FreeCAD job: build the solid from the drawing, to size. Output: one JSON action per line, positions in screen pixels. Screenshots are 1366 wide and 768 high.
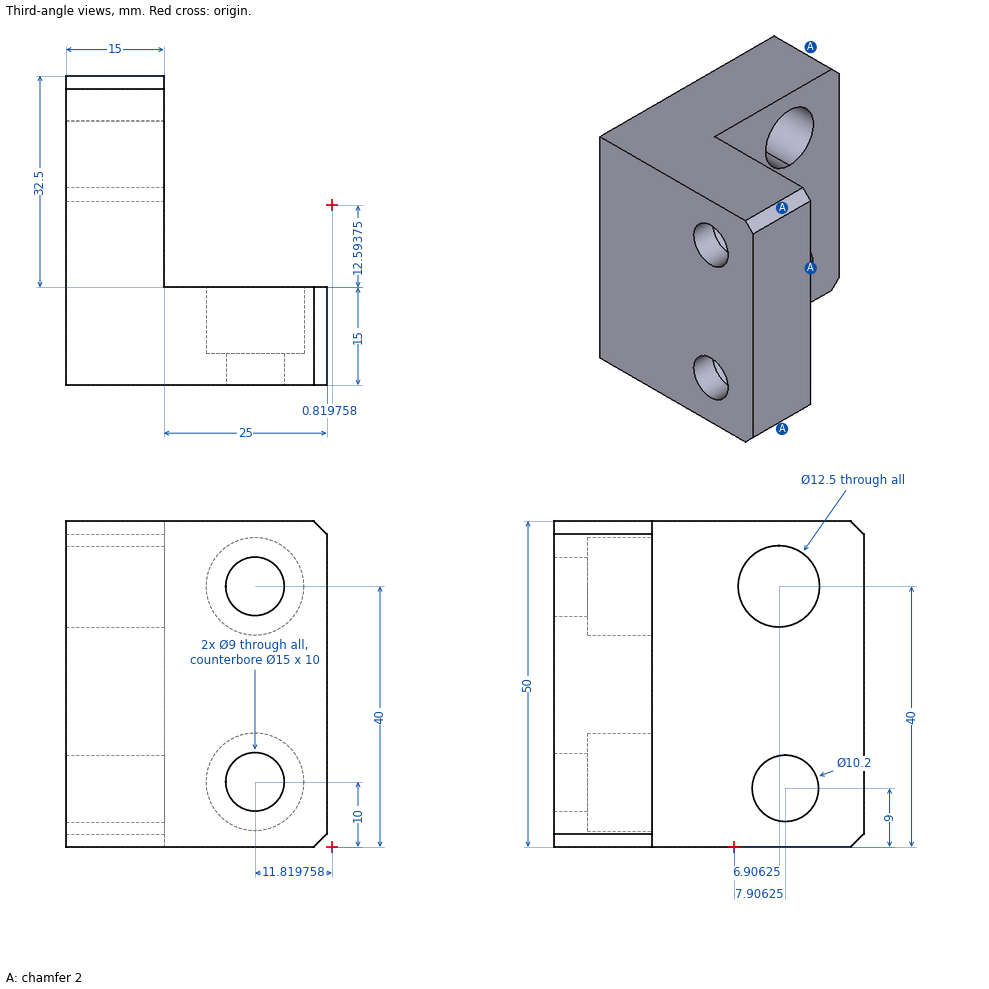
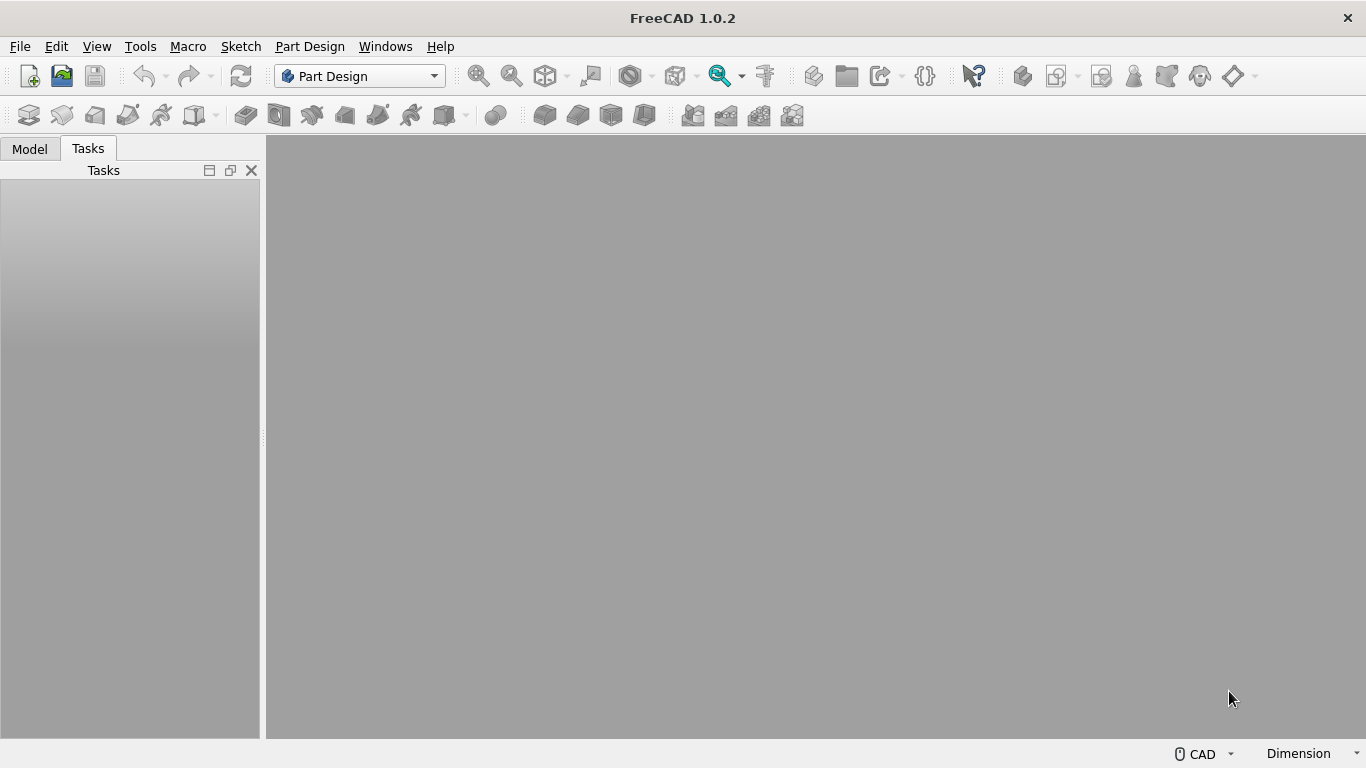
{"action": "left_click", "coordinate": [29, 76]}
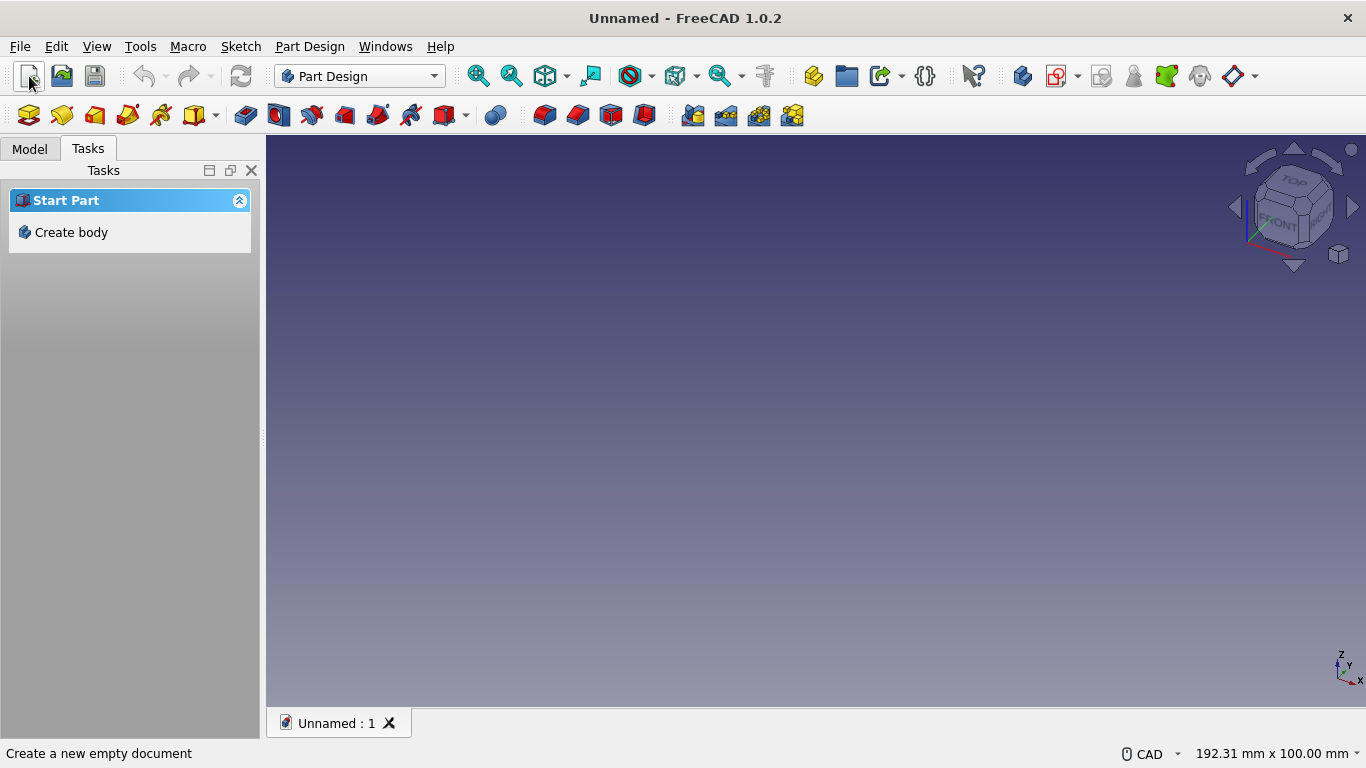
{"action": "left_click", "coordinate": [1056, 76]}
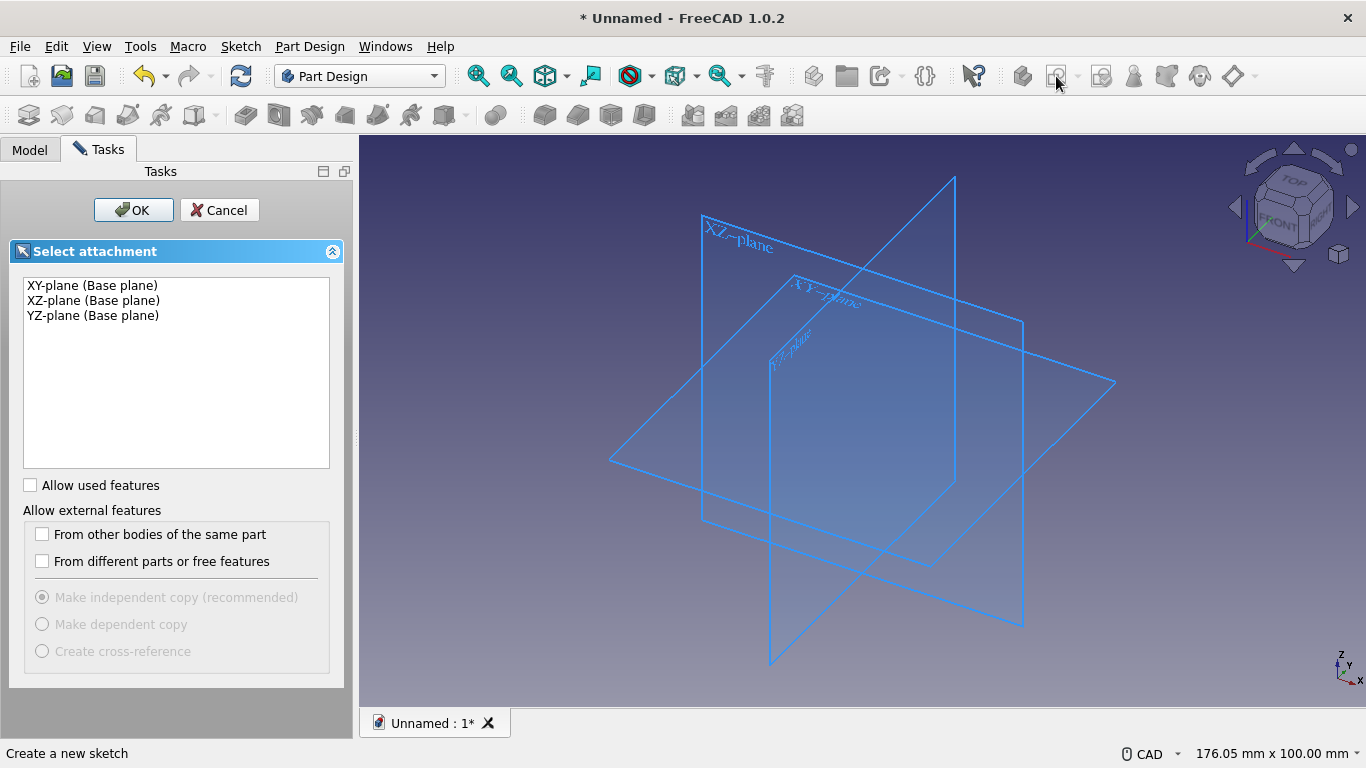
{"action": "left_click", "coordinate": [84, 286]}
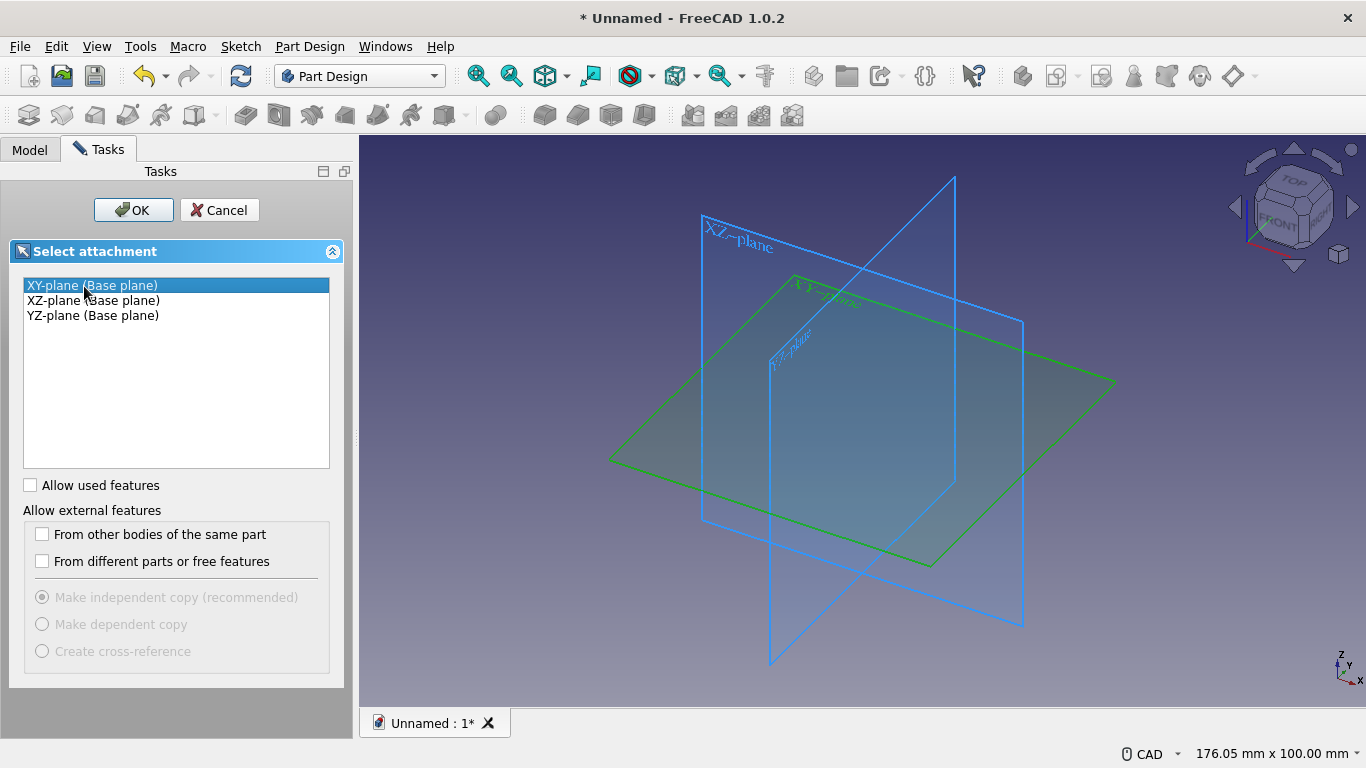
{"action": "left_click", "coordinate": [134, 210]}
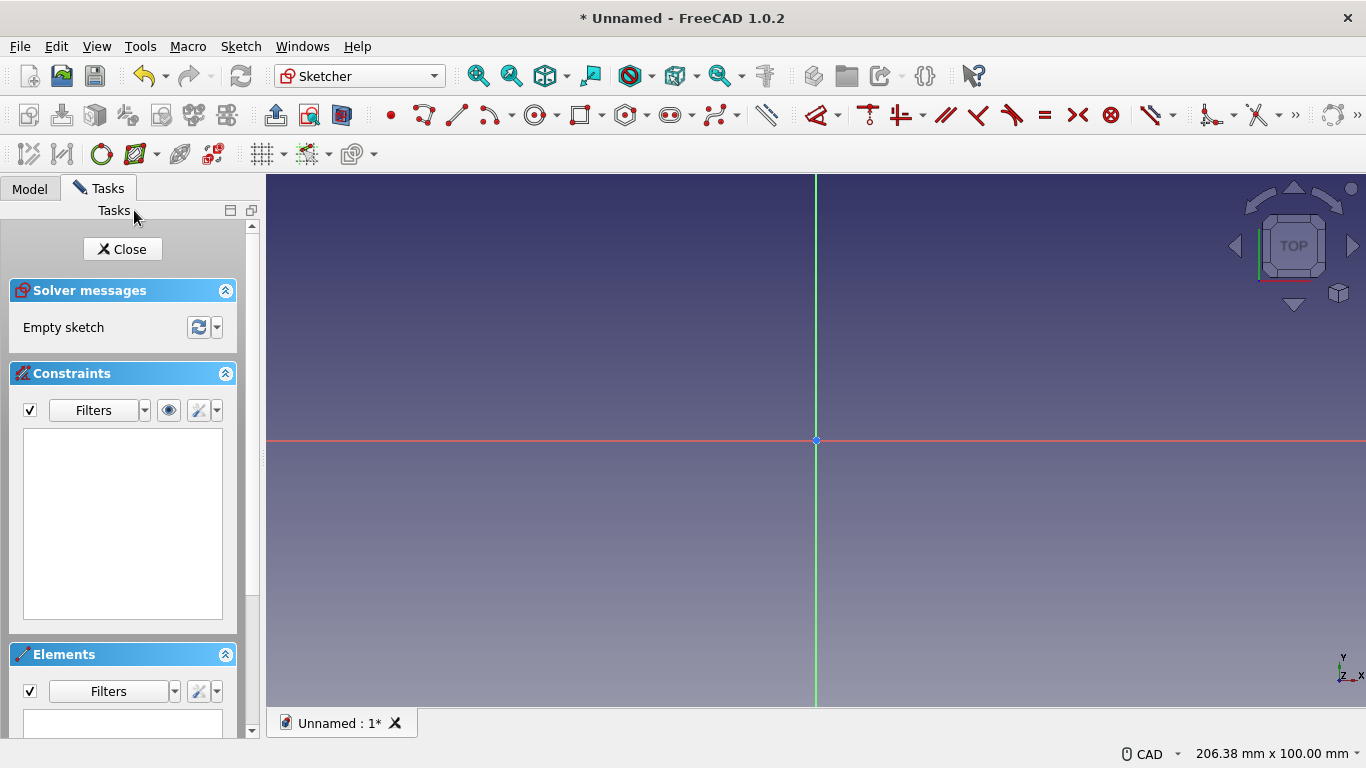
{"action": "left_click", "coordinate": [424, 116]}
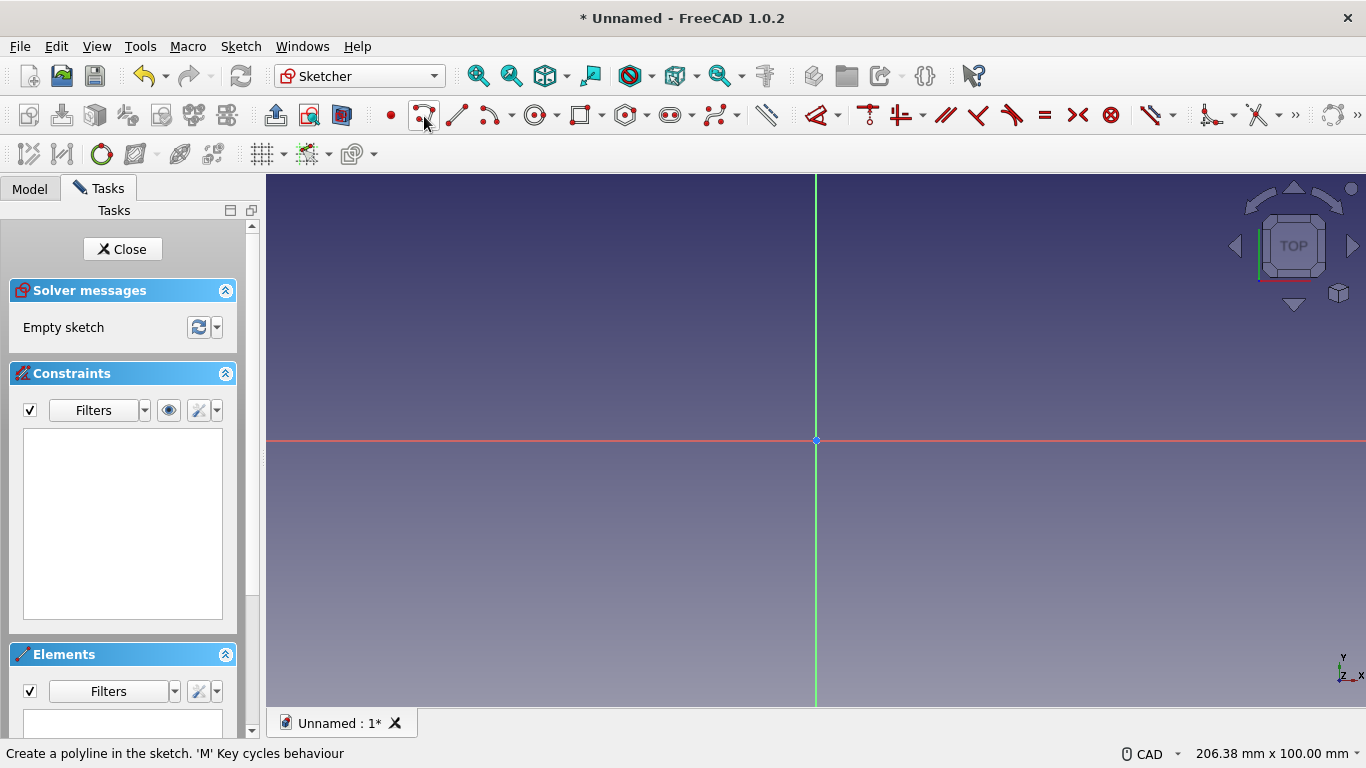
{"action": "scroll", "coordinate": [812, 508], "scroll_direction": "up", "scroll_amount": 7}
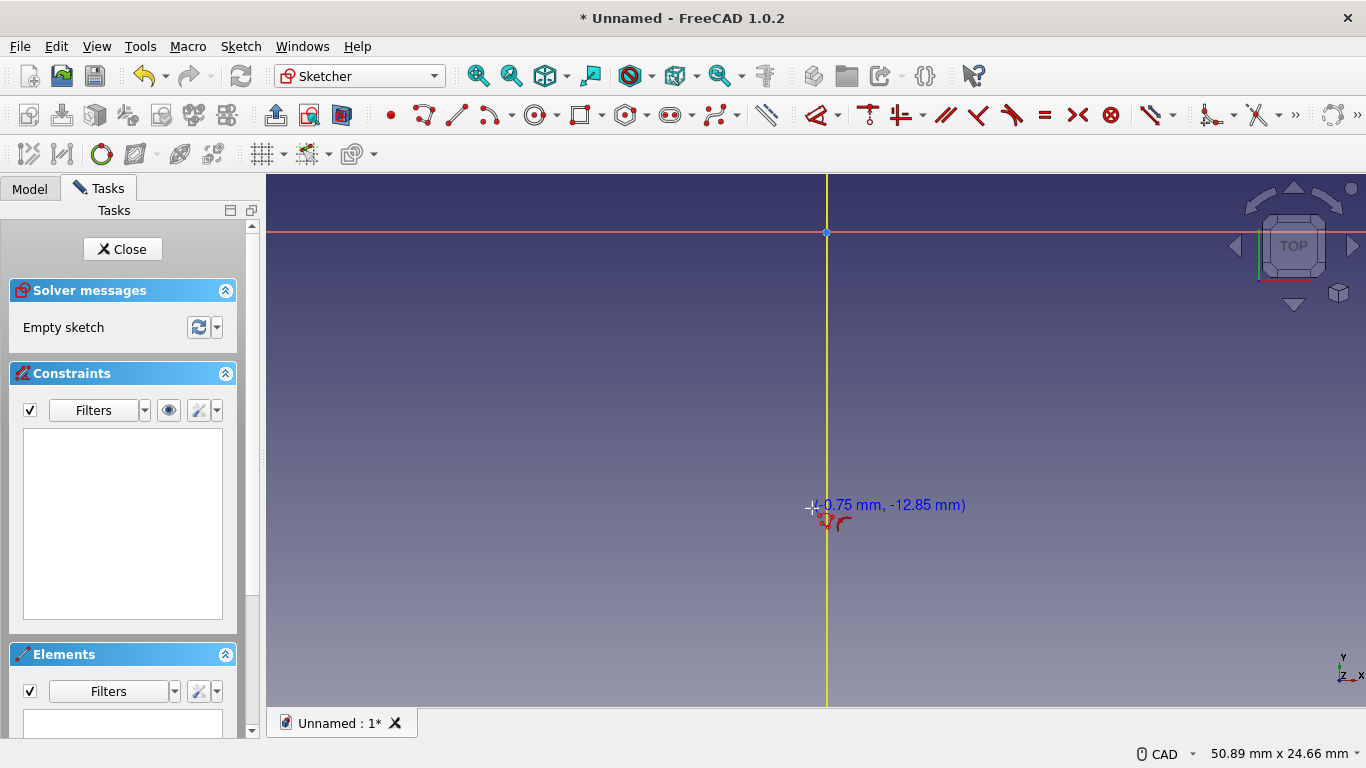
{"action": "left_click", "coordinate": [809, 505]}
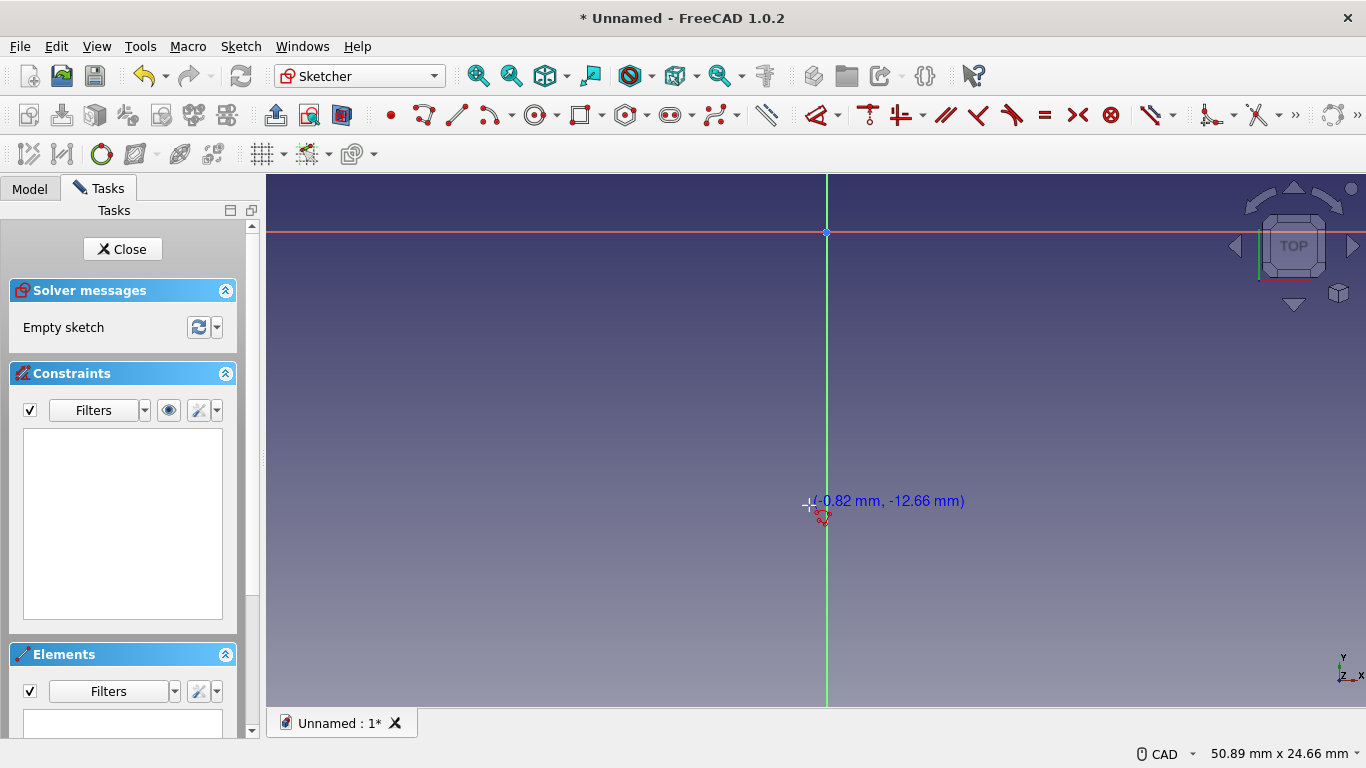
{"action": "scroll", "coordinate": [904, 494], "scroll_direction": "down", "scroll_amount": 6}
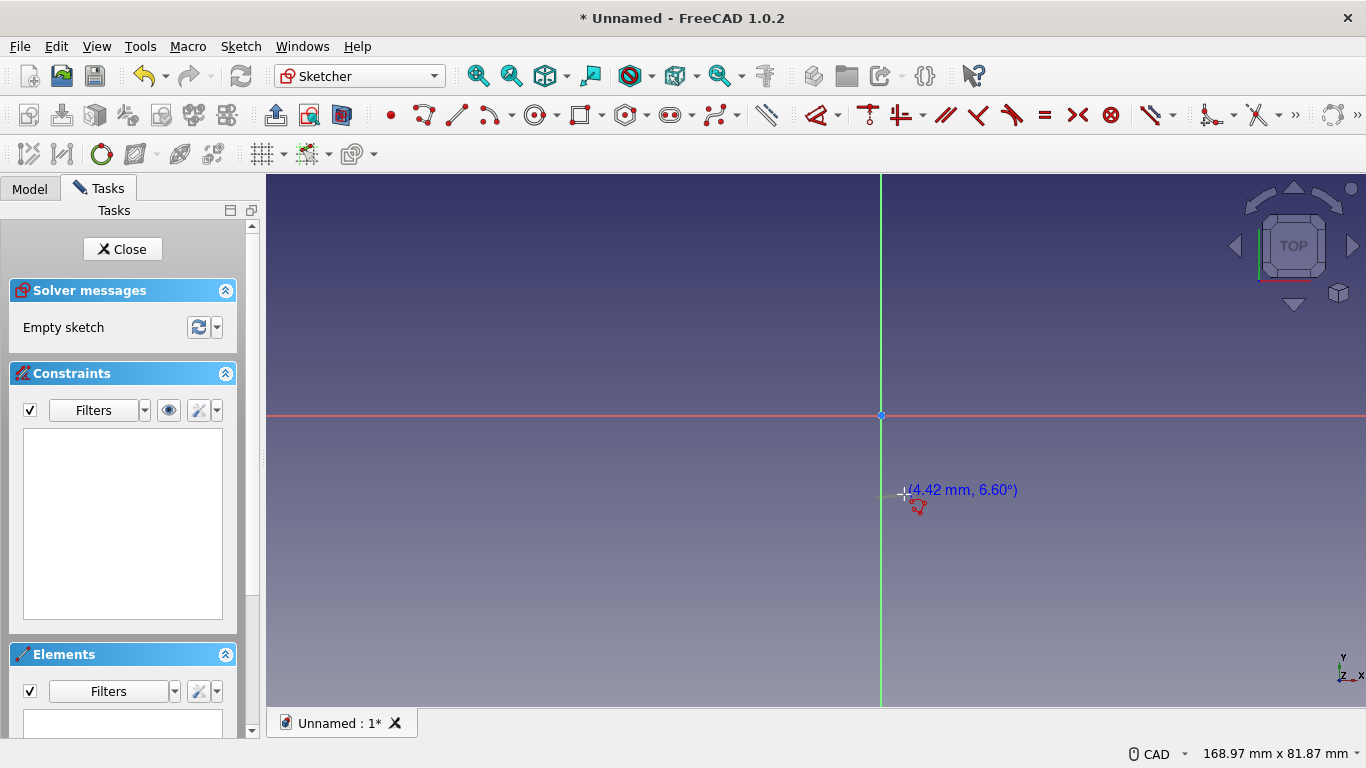
{"action": "left_click", "coordinate": [713, 498]}
{"action": "left_click", "coordinate": [713, 286]}
{"action": "left_click", "coordinate": [615, 286]}
{"action": "left_click", "coordinate": [615, 595]}